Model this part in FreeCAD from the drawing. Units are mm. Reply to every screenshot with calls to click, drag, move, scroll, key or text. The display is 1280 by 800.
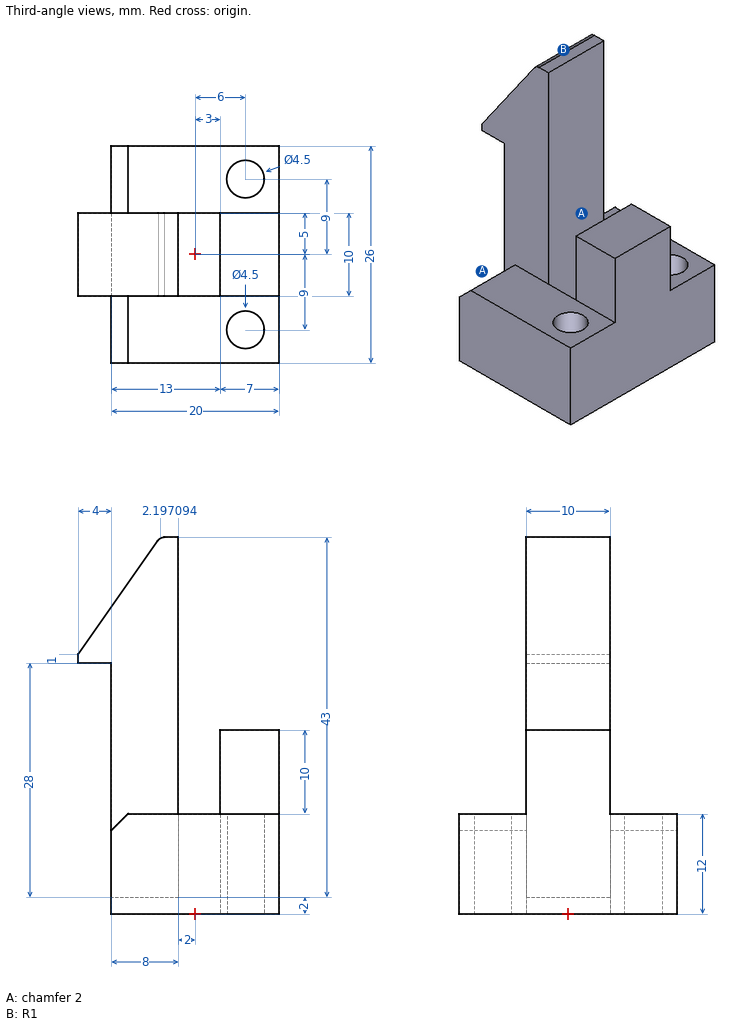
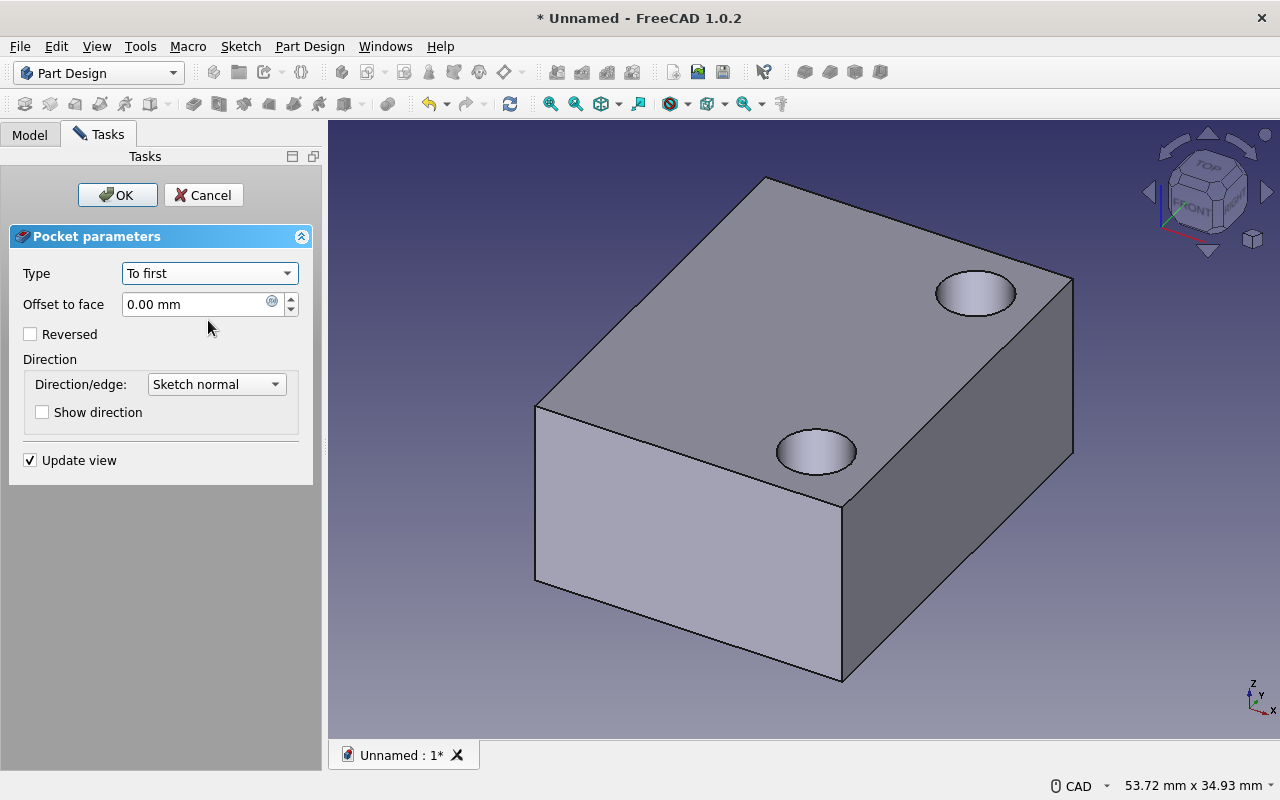
click(118, 195)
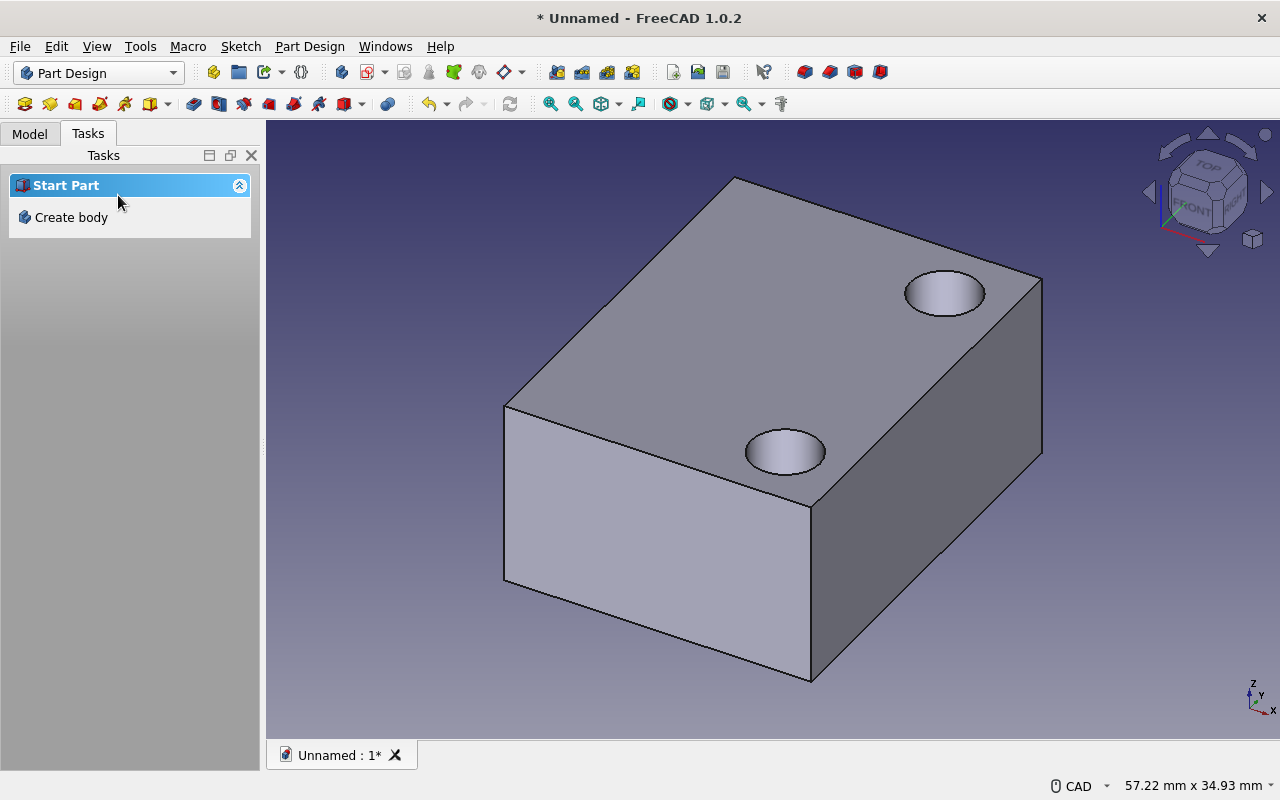
click(773, 341)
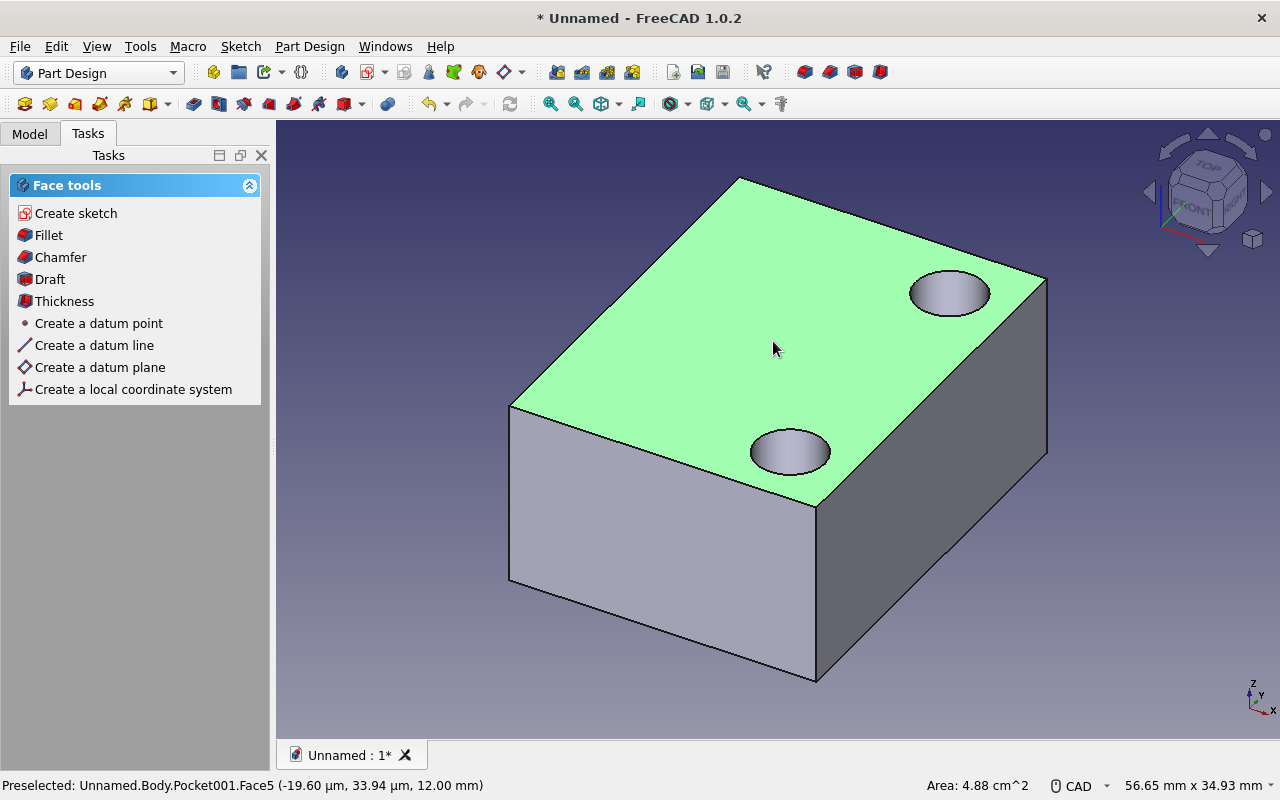
click(366, 72)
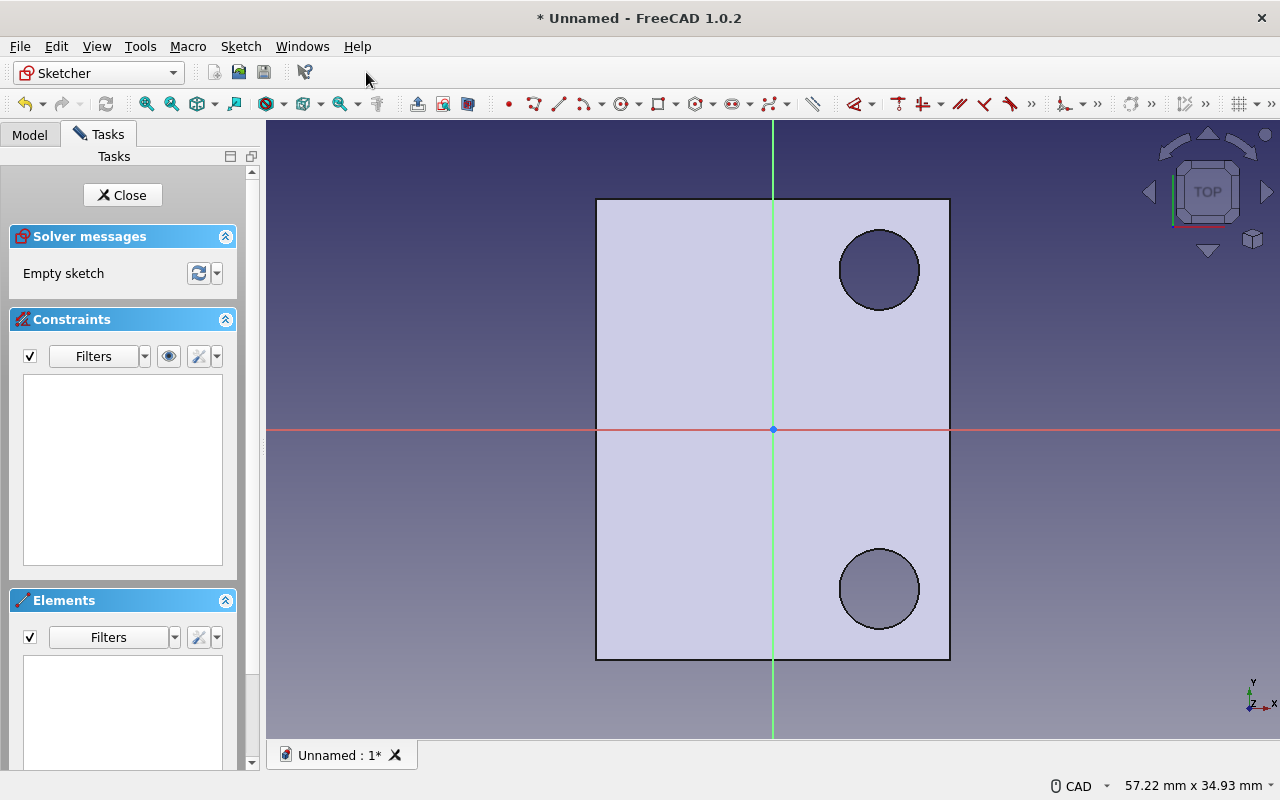
scroll(990, 430, up, 4)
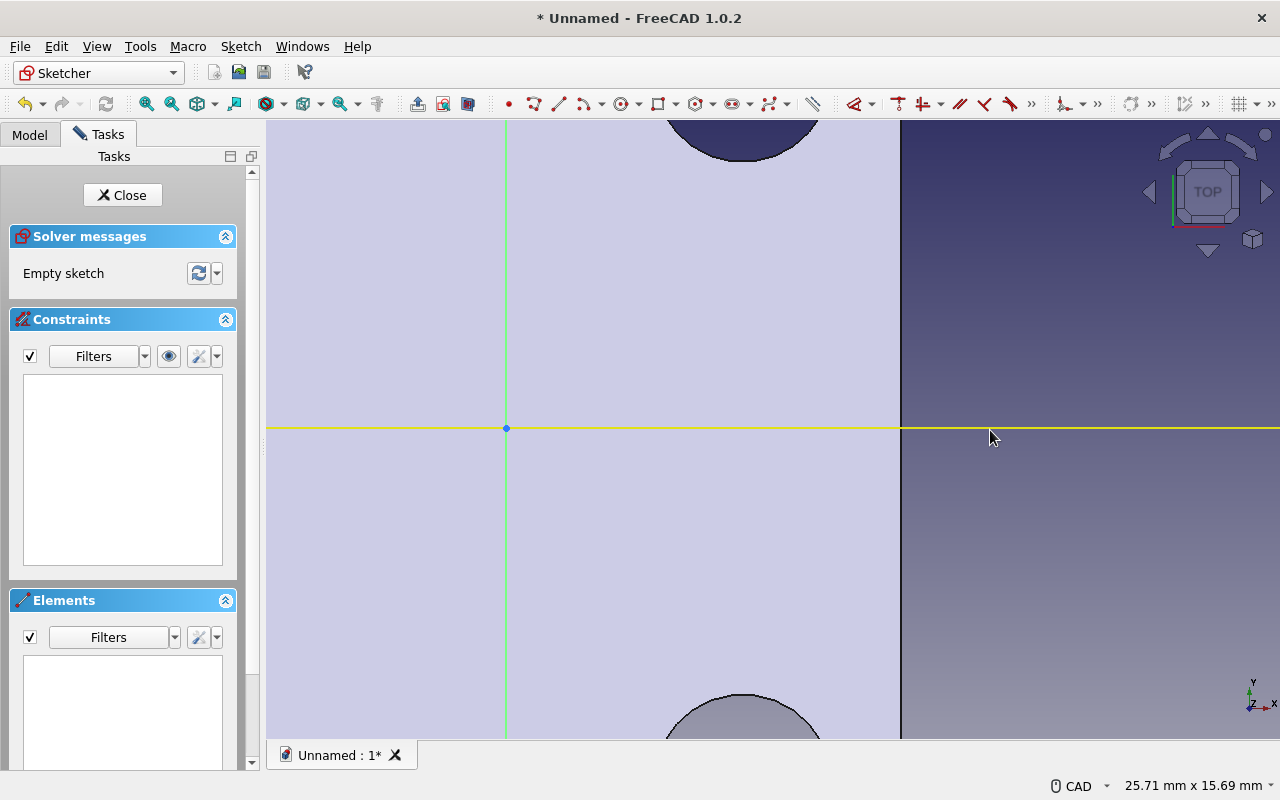
click(658, 104)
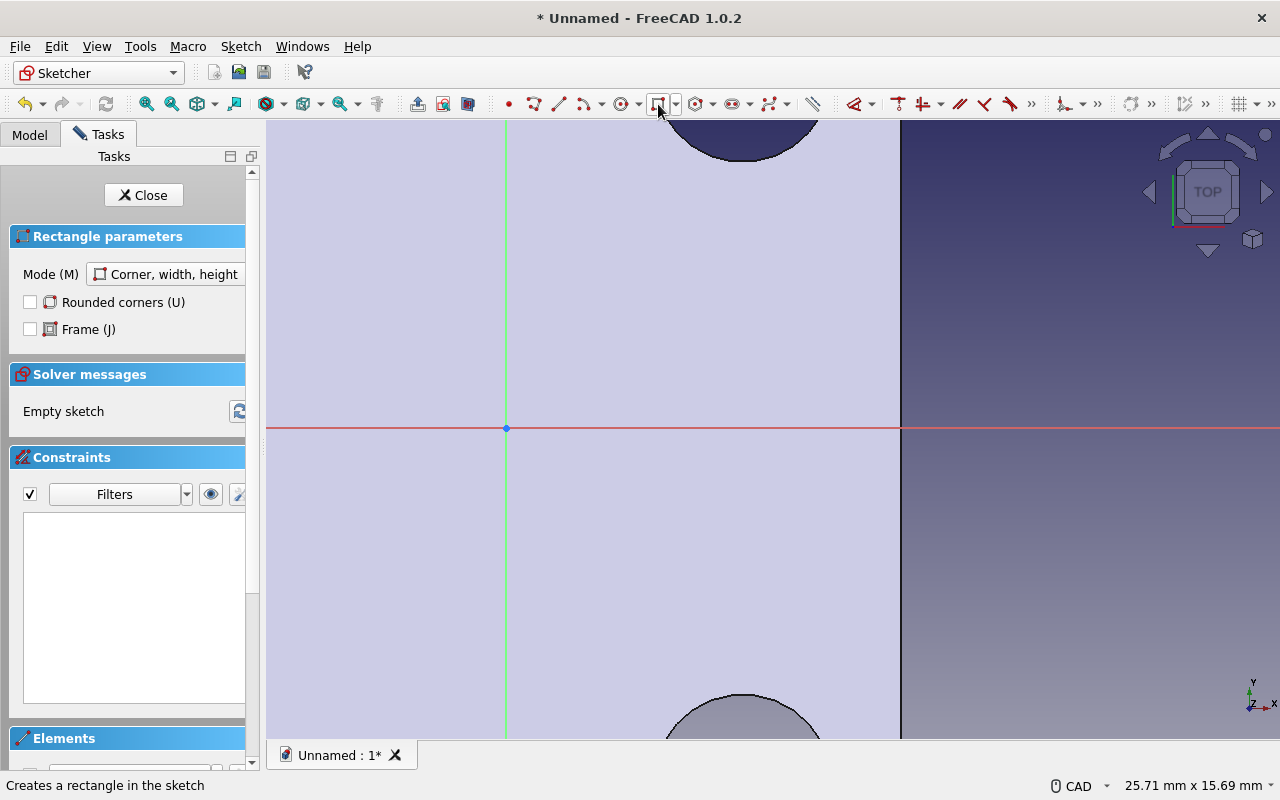
click(625, 231)
click(901, 625)
key(Escape)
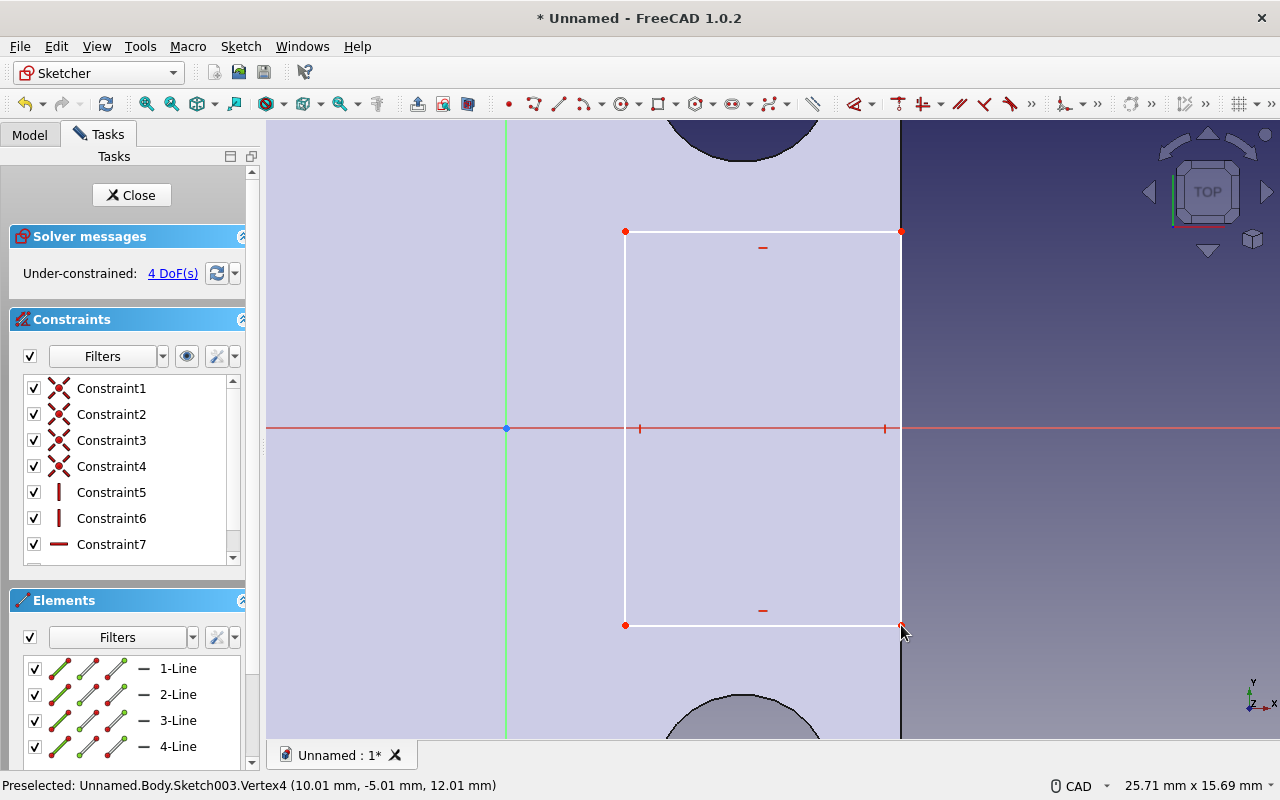
key(d)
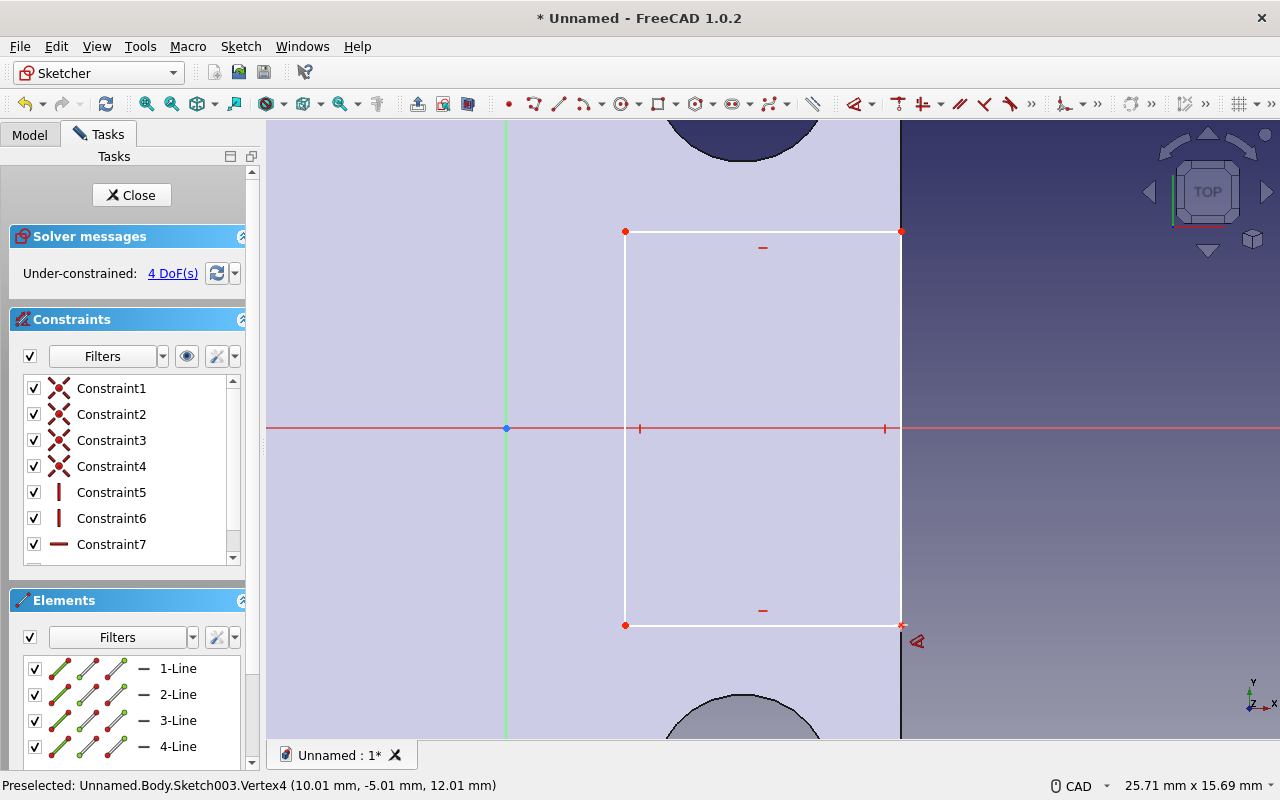
click(708, 626)
click(763, 660)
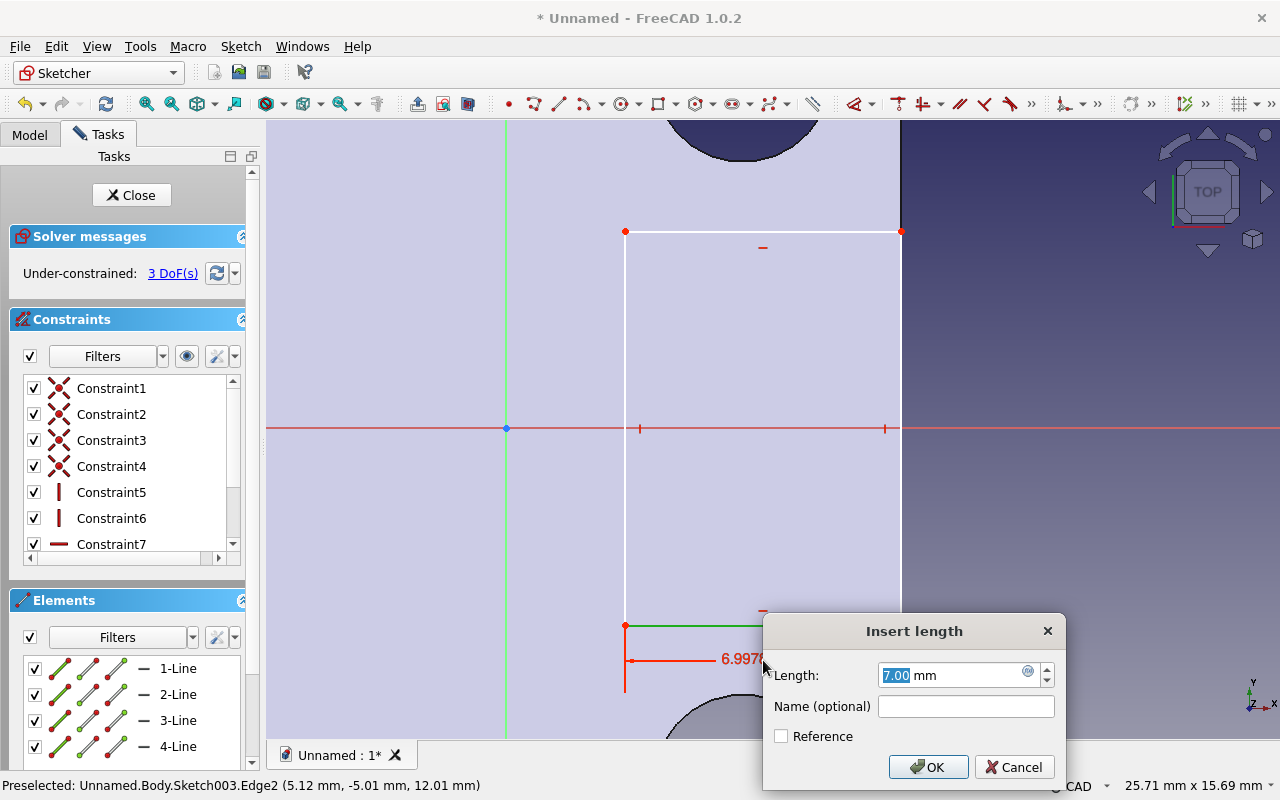
text(7)
key(Return)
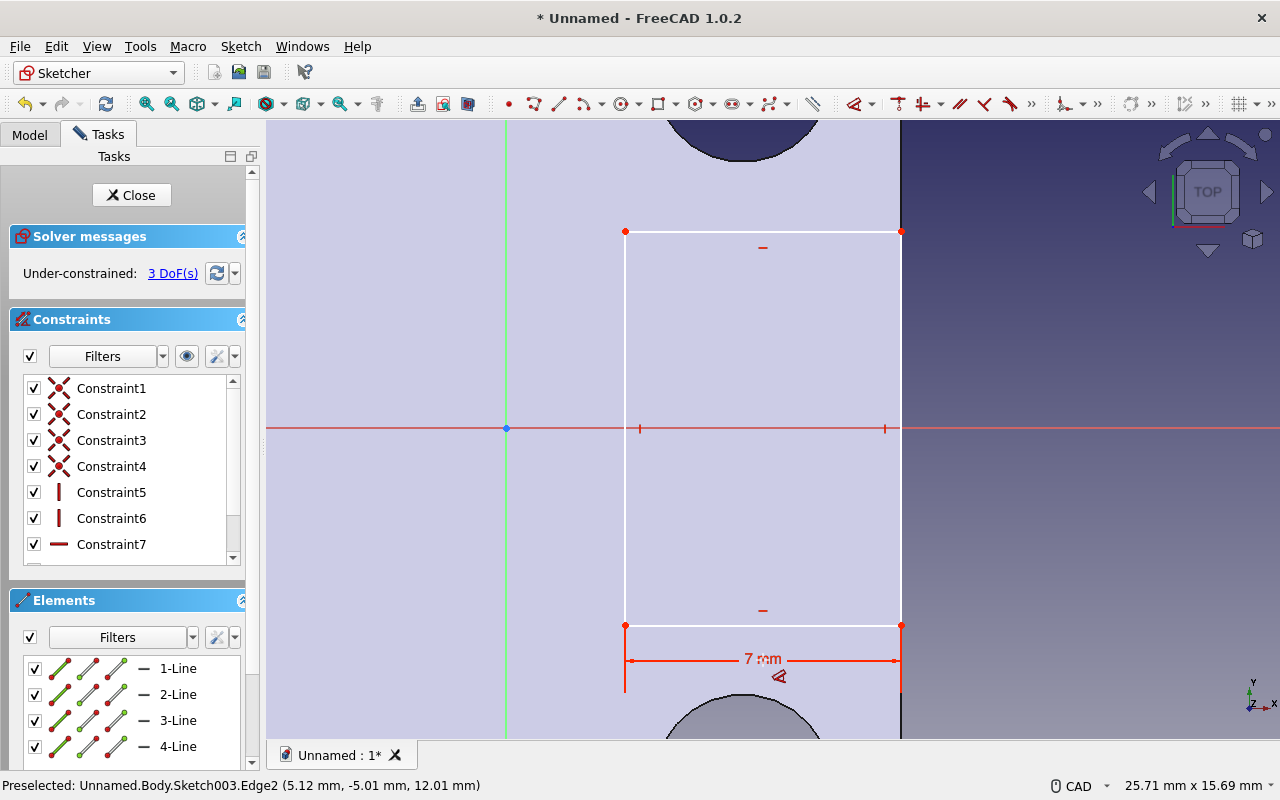
click(625, 350)
click(591, 338)